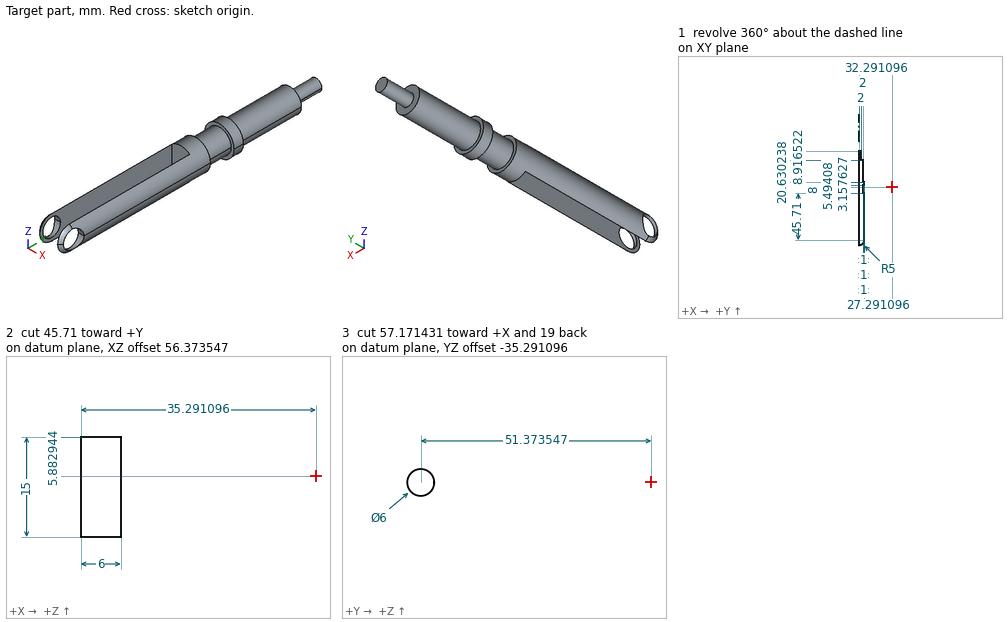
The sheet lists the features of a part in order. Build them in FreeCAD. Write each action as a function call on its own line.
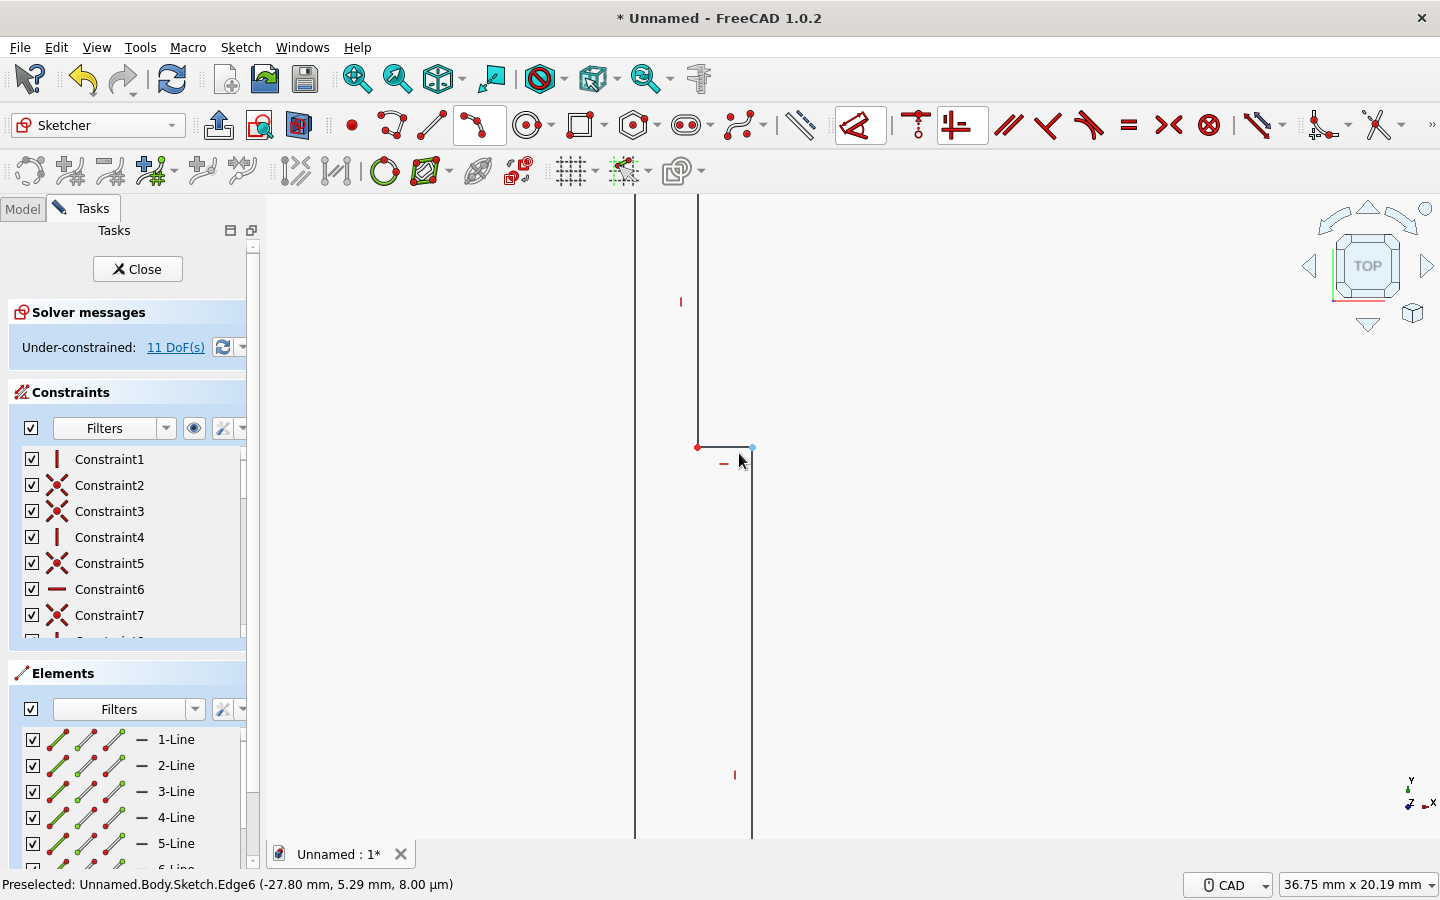
click(736, 447)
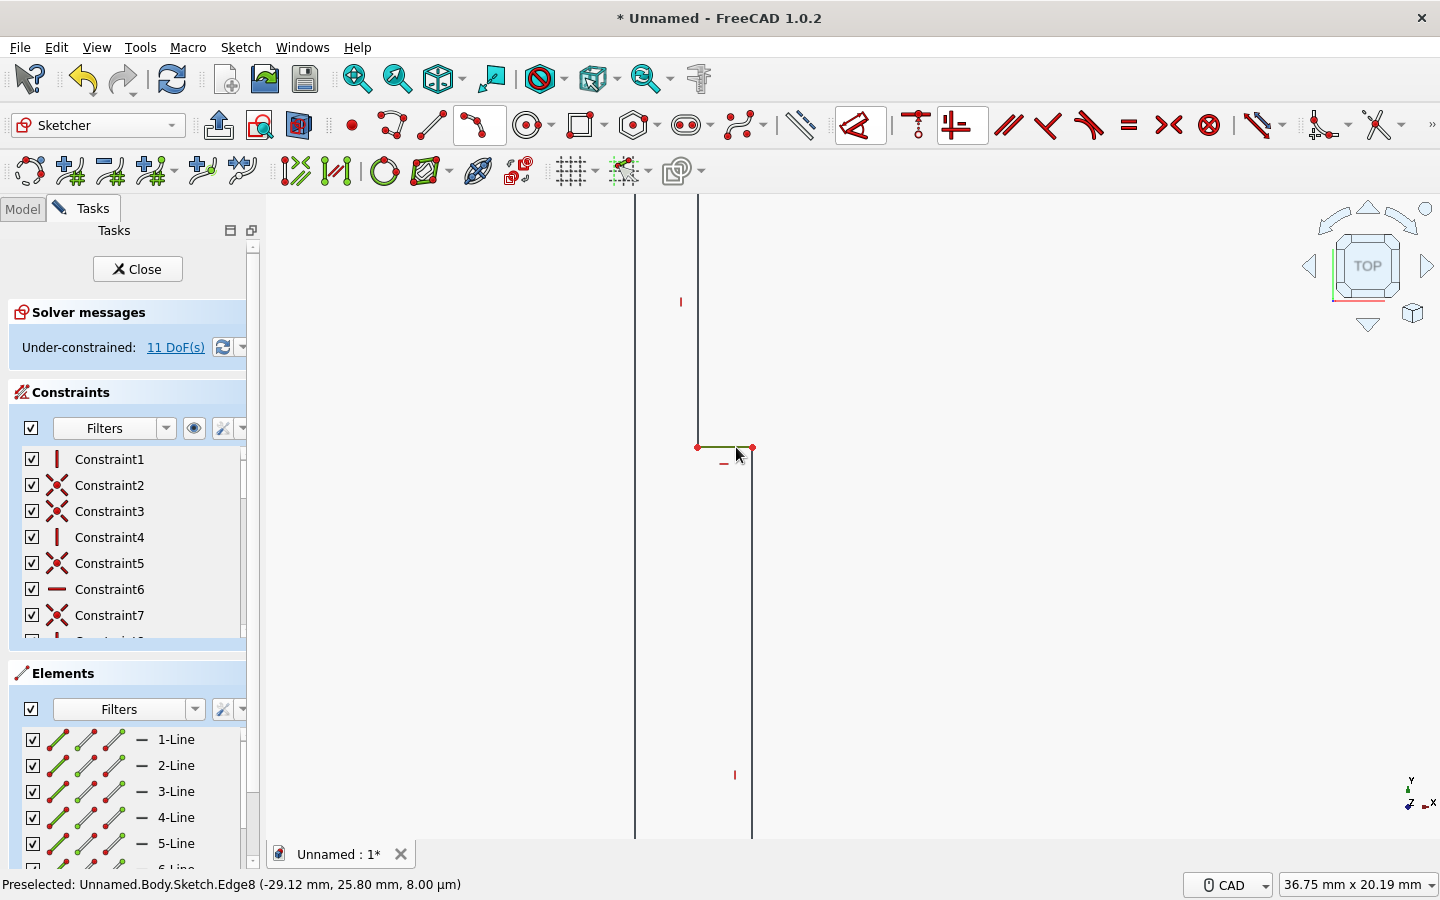
key(l)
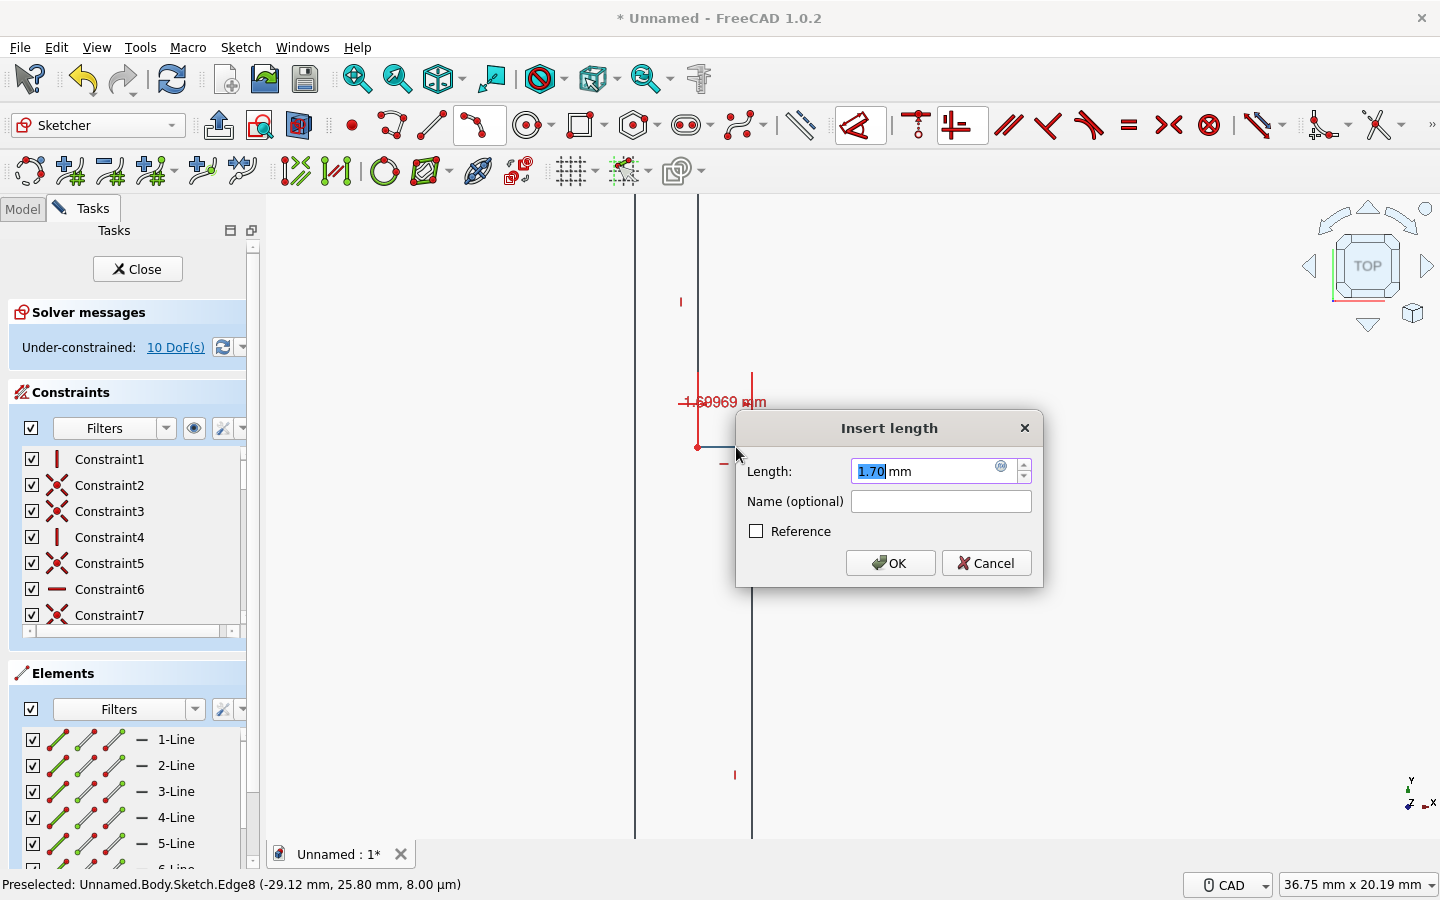
text(2)
key(Return)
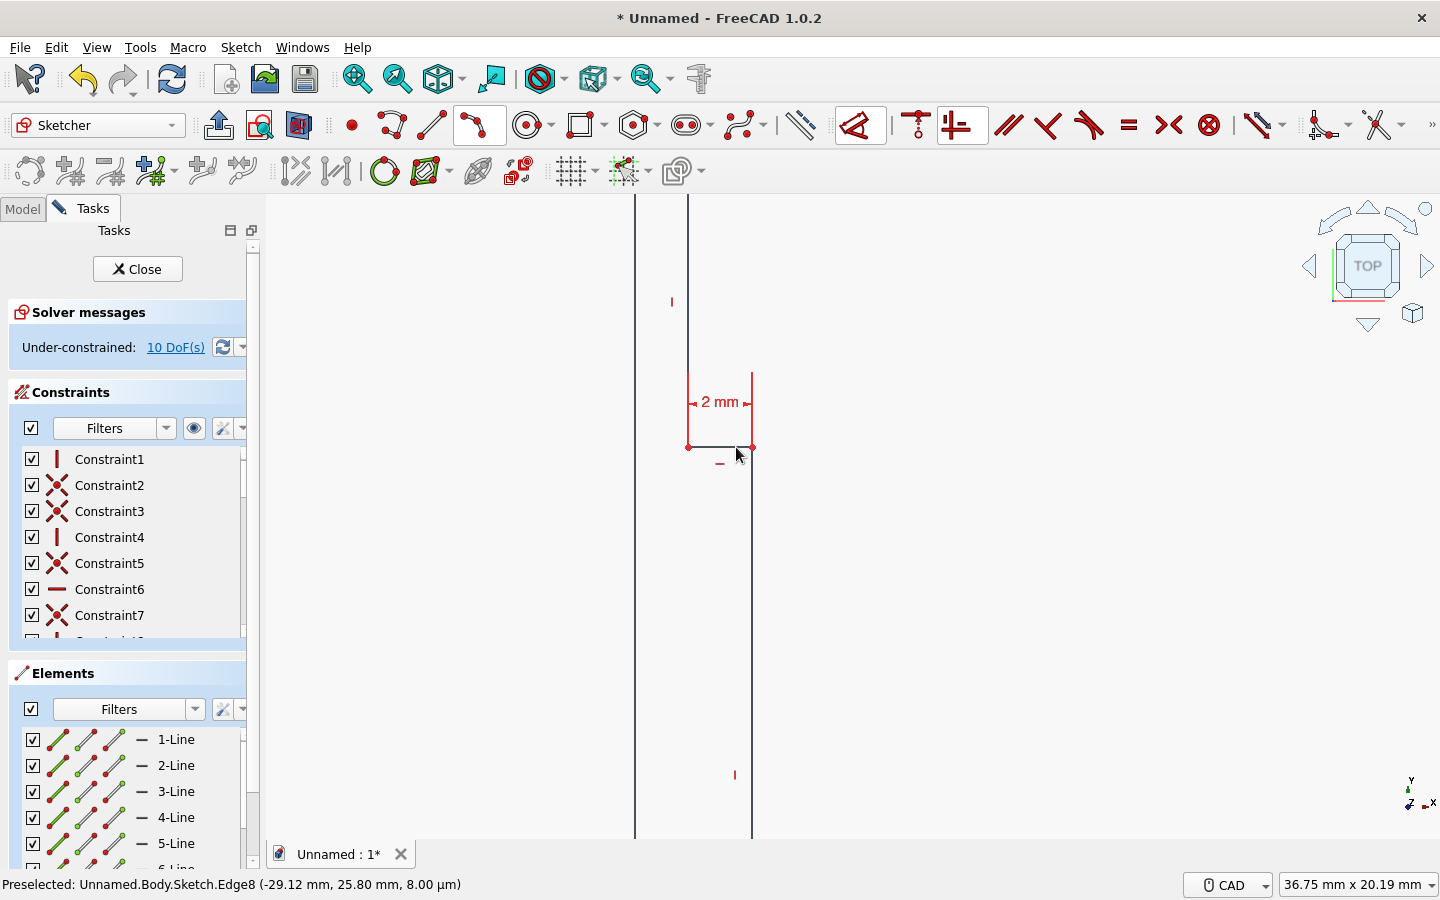
scroll(739, 453, down, 11)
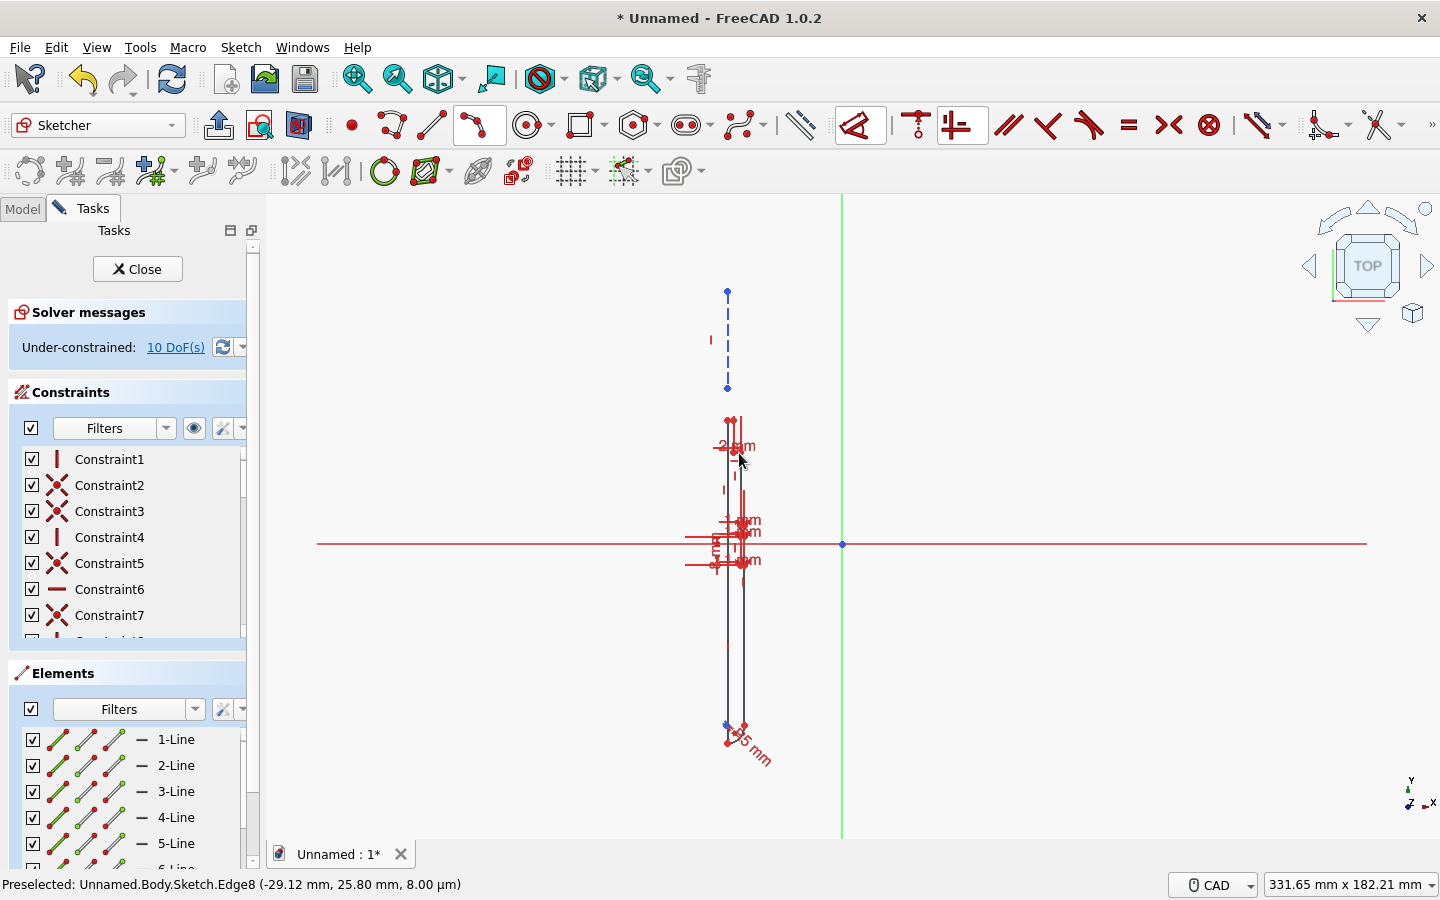
scroll(732, 420, up, 11)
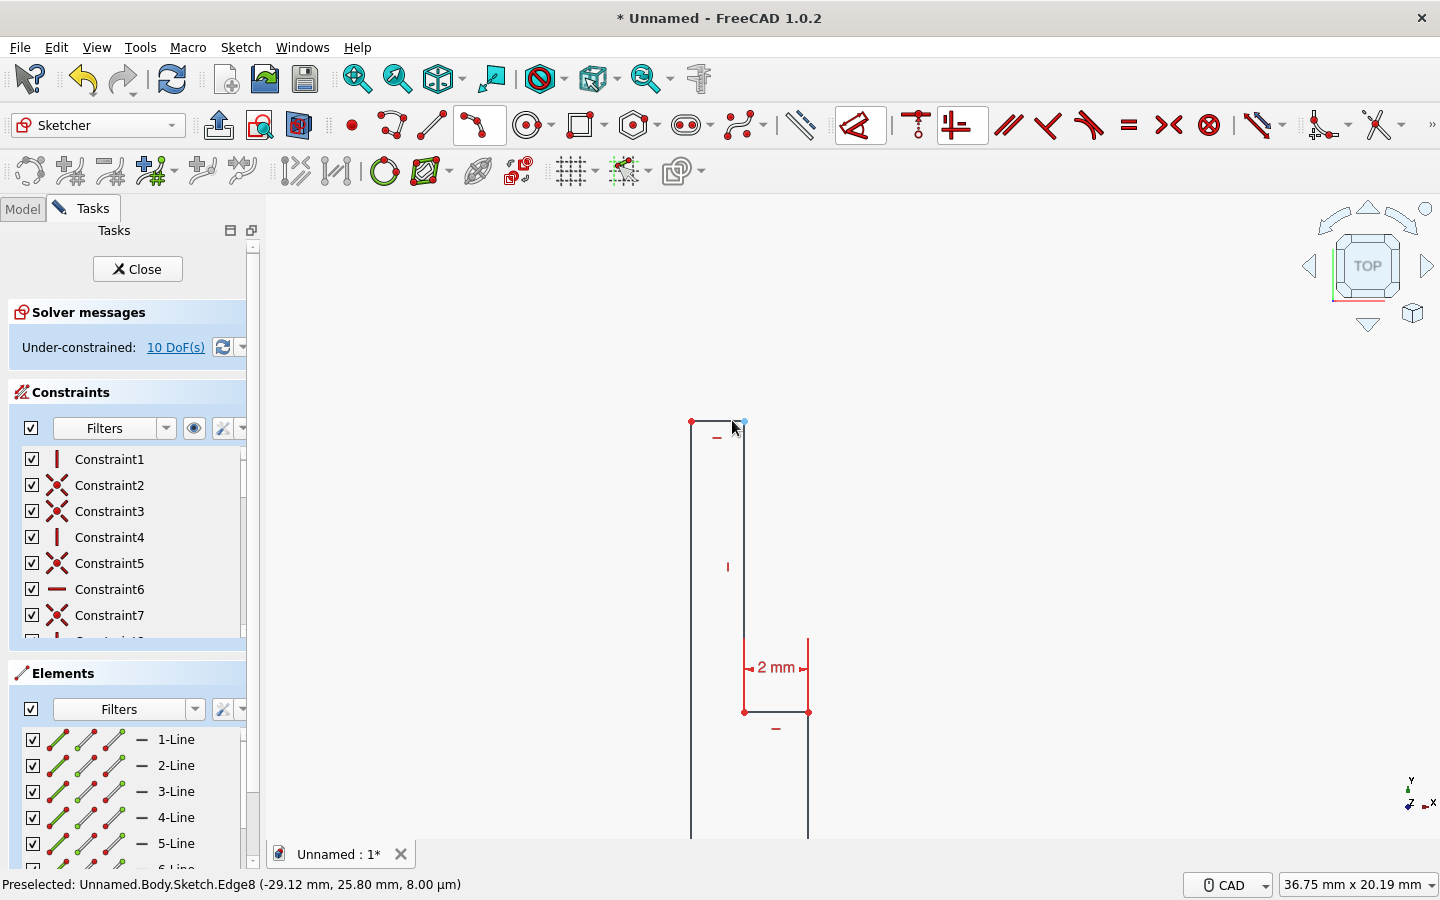
click(728, 421)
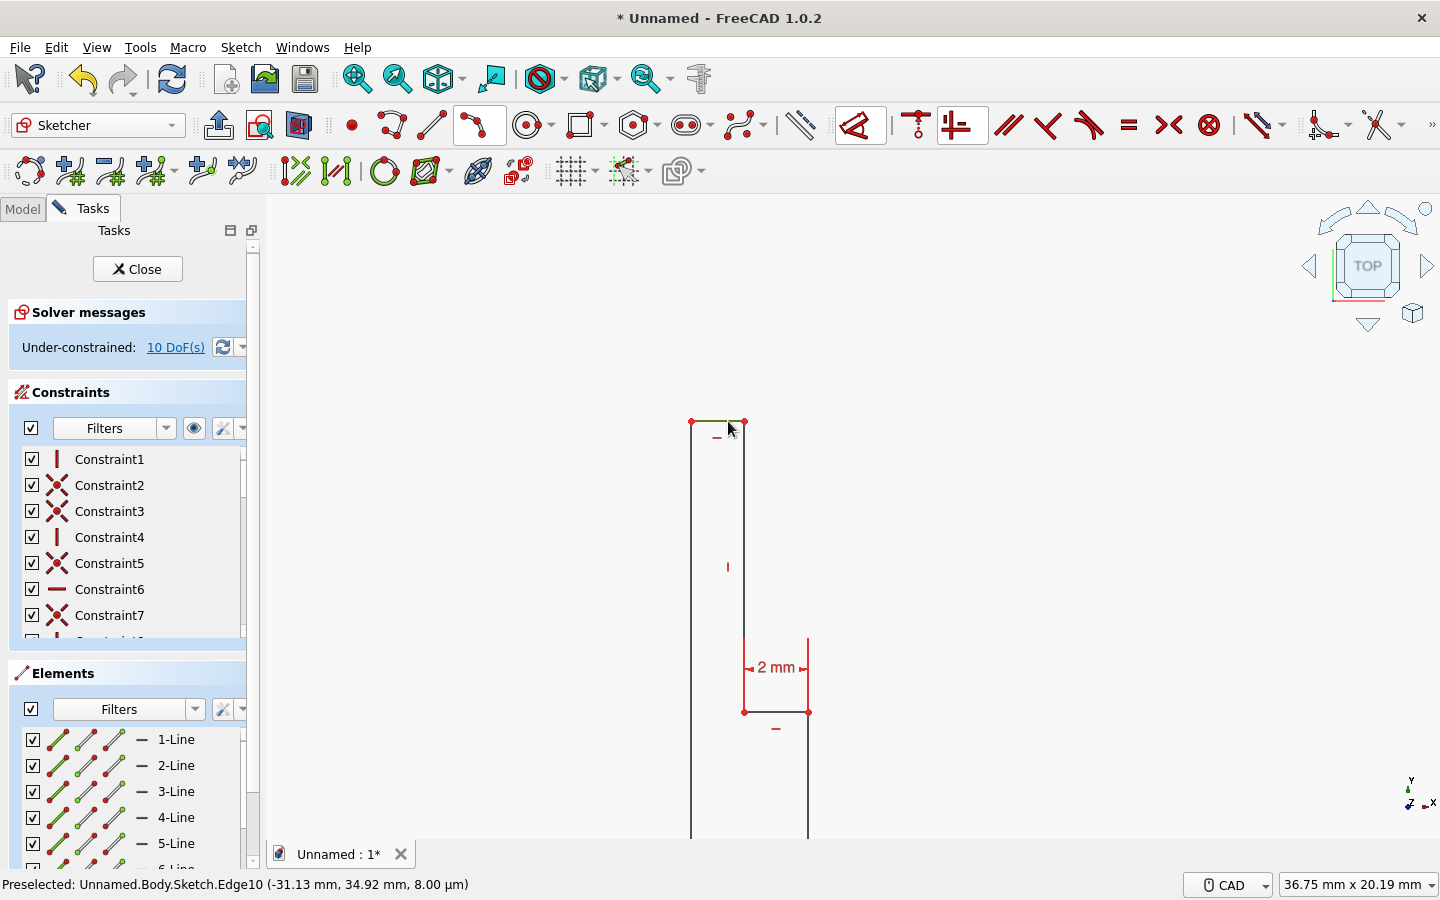
click(880, 126)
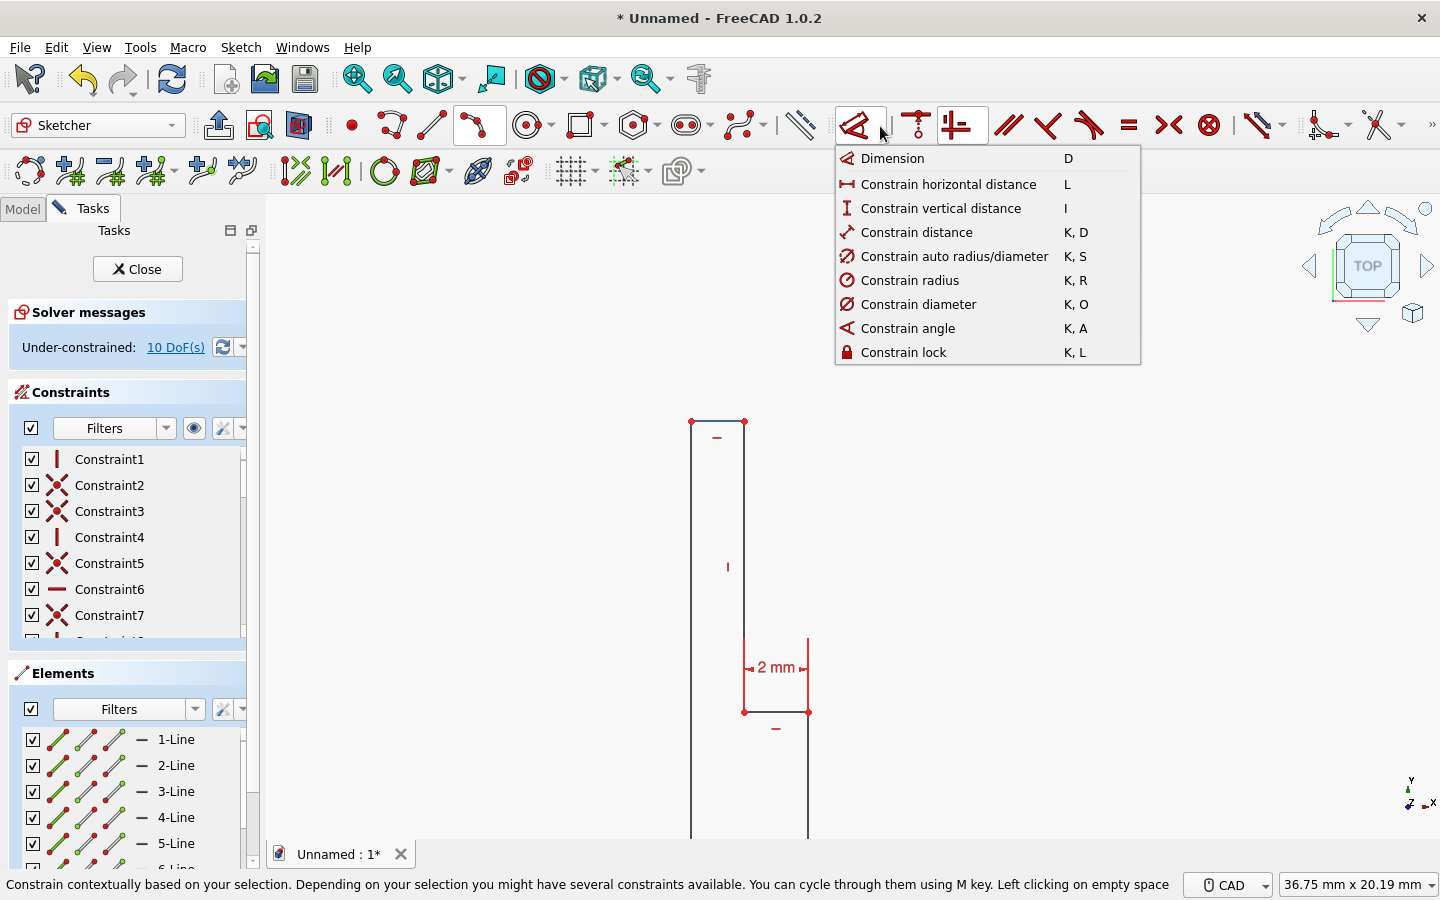
click(988, 184)